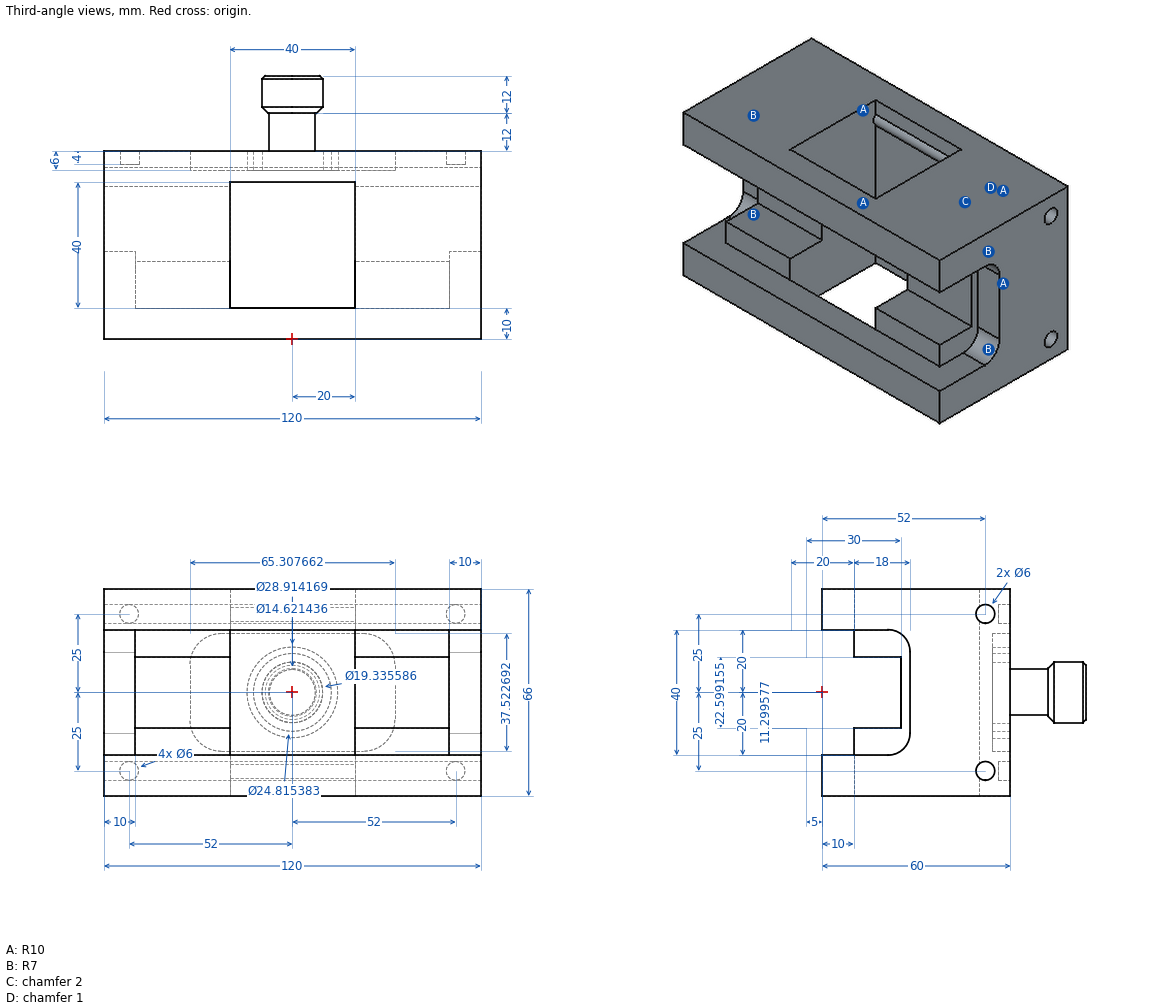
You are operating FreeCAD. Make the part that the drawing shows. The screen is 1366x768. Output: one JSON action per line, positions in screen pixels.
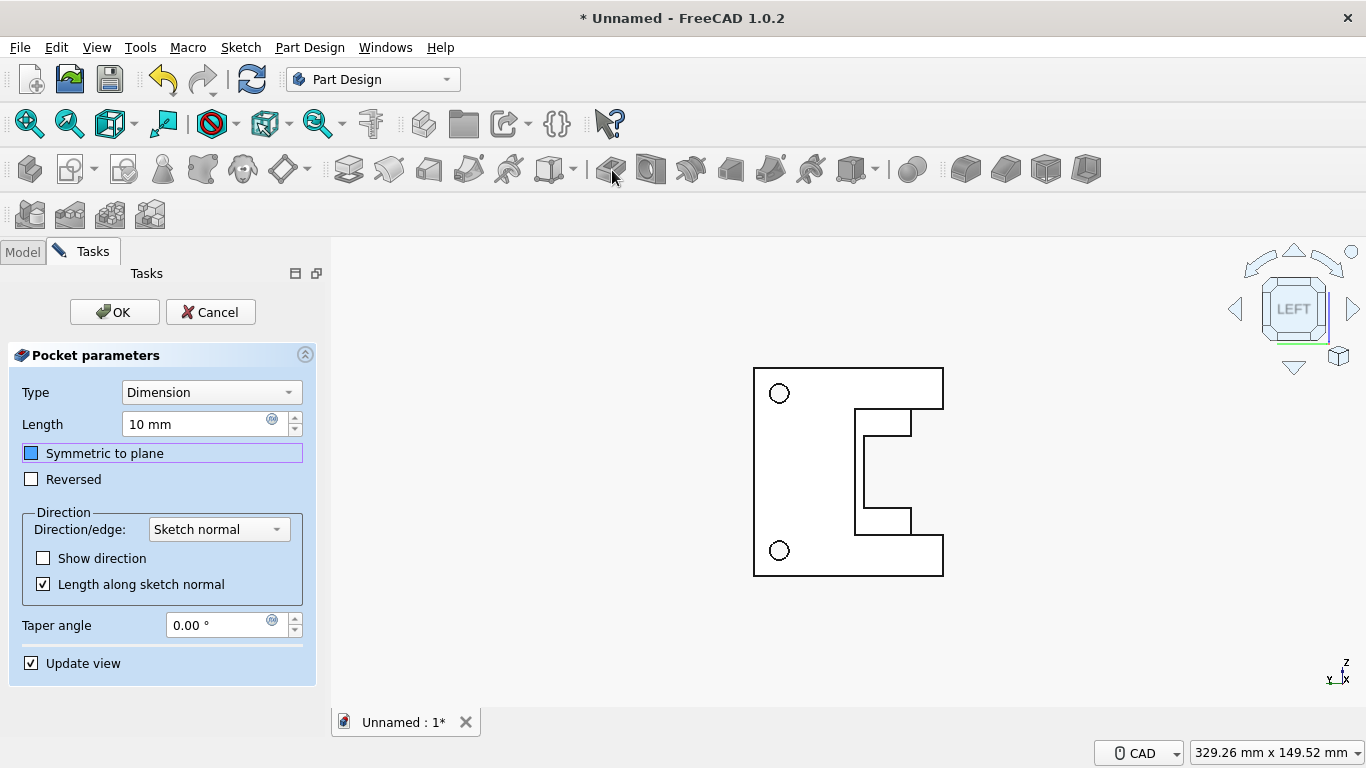
{"action": "left_click", "coordinate": [115, 312]}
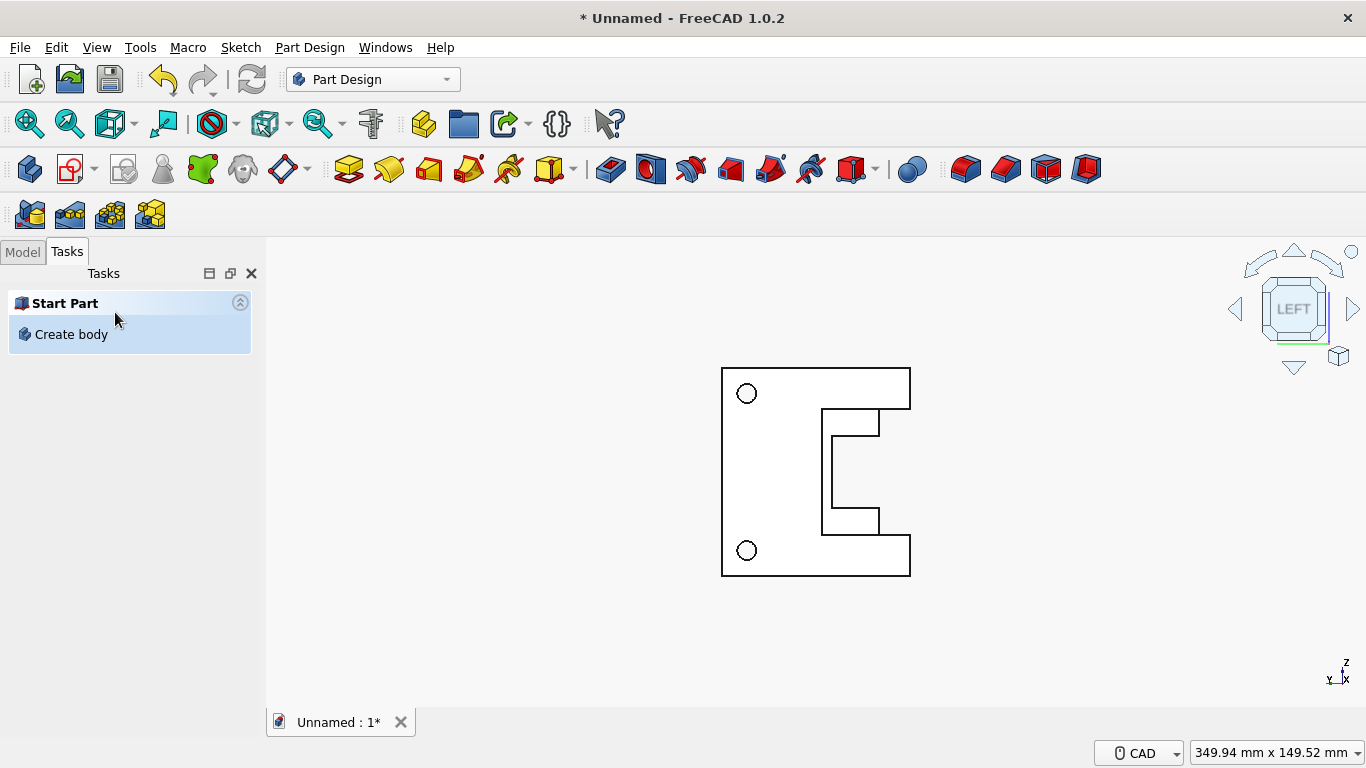
{"action": "left_click", "coordinate": [30, 124]}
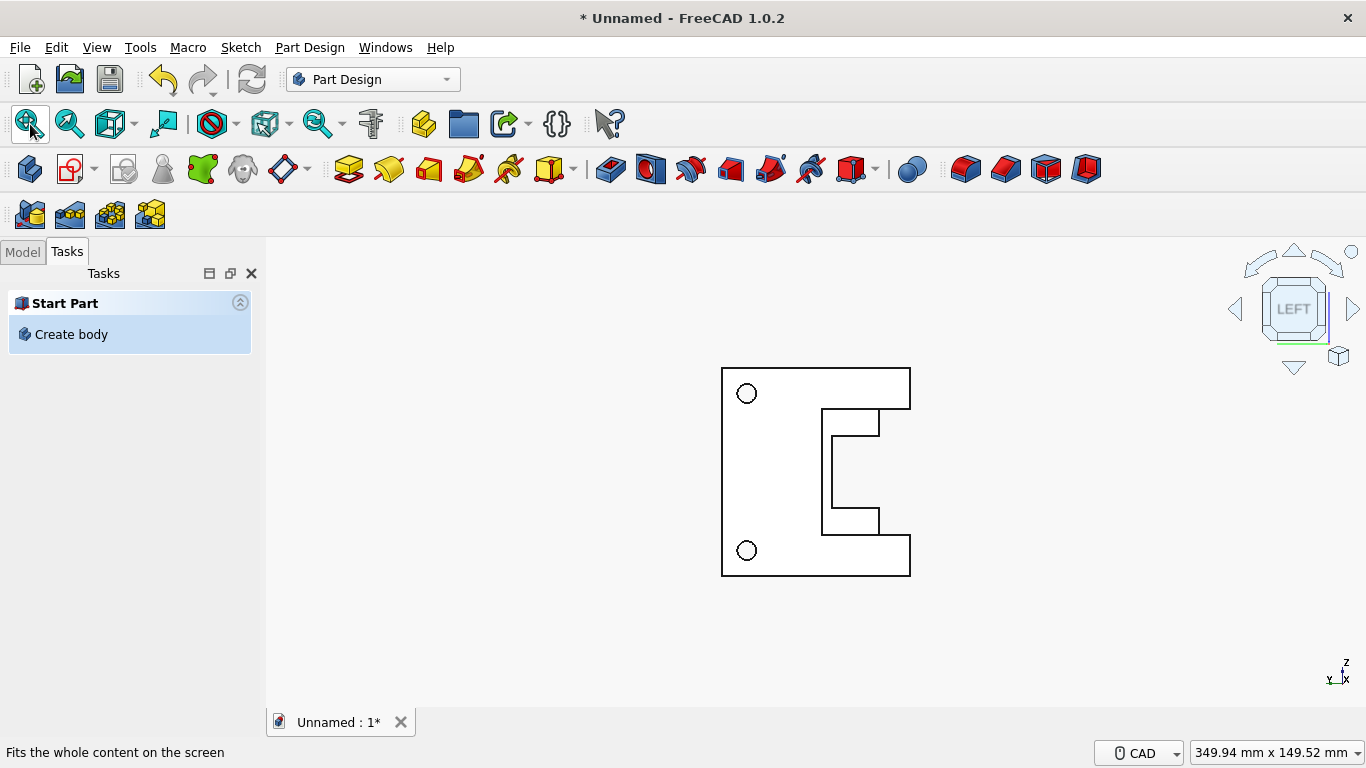
{"action": "key", "text": "4"}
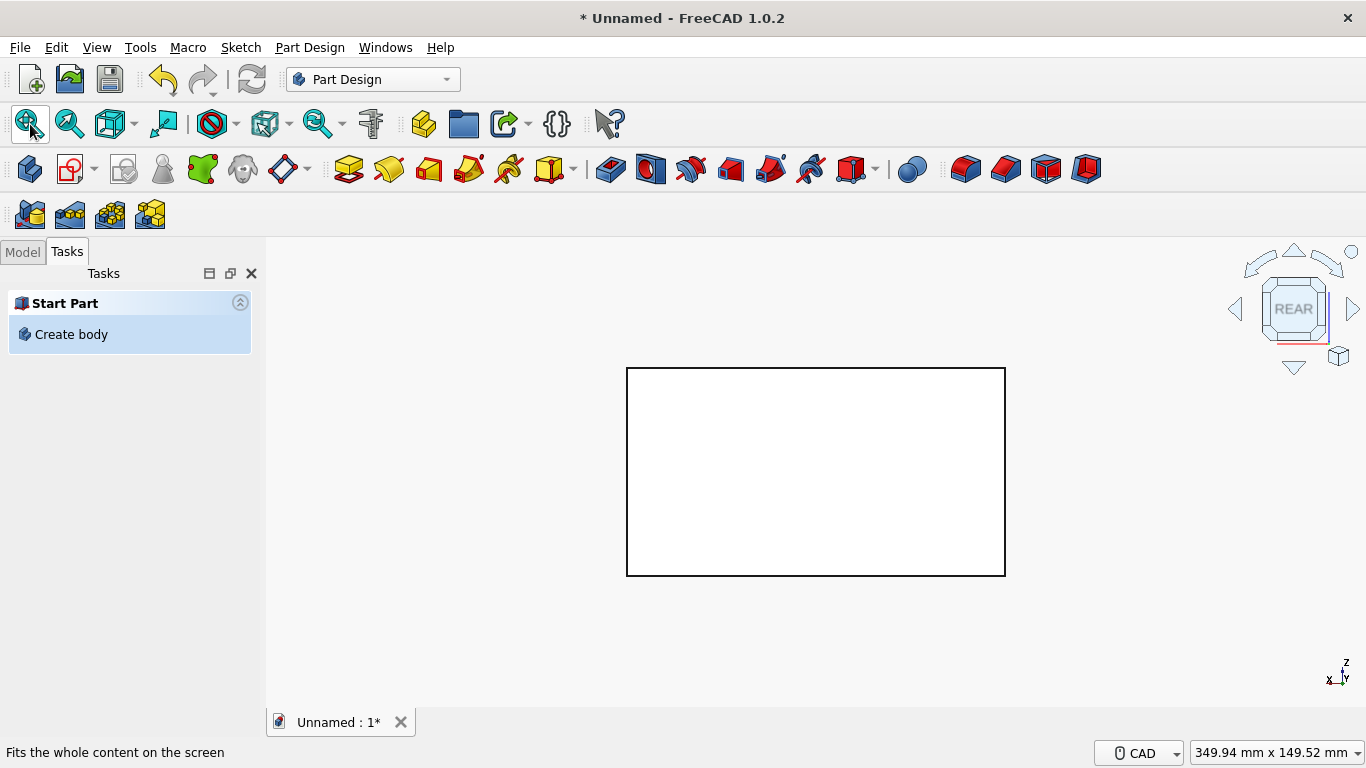
{"action": "left_click", "coordinate": [30, 124]}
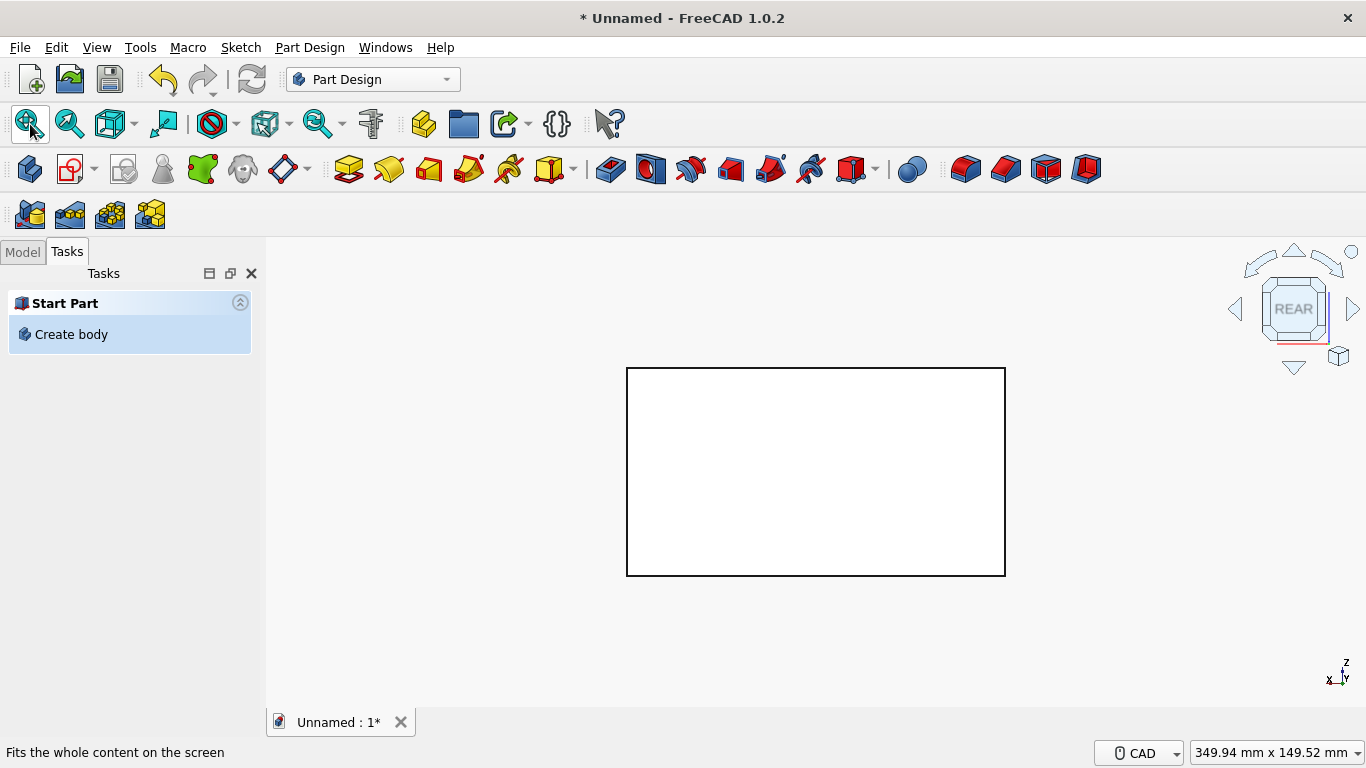
{"action": "left_click", "coordinate": [762, 471]}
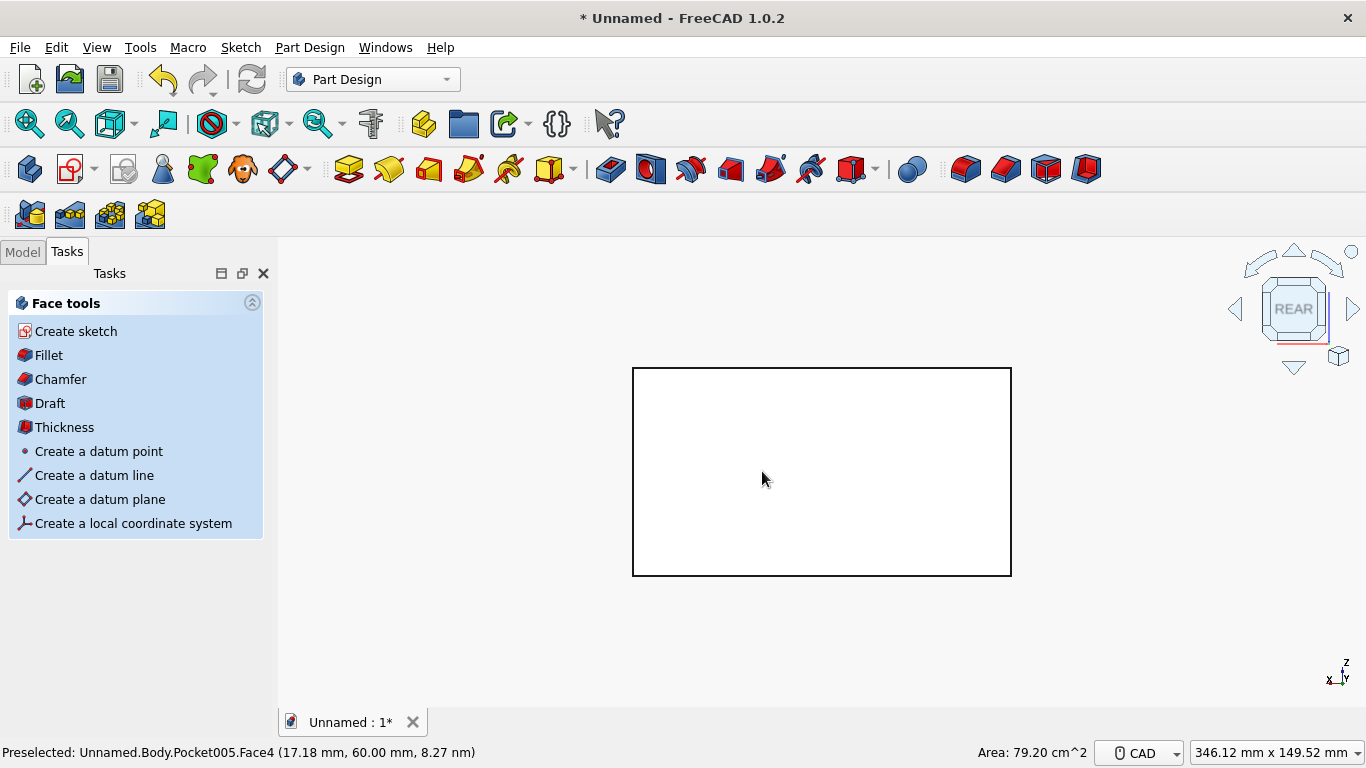
{"action": "left_click", "coordinate": [70, 170]}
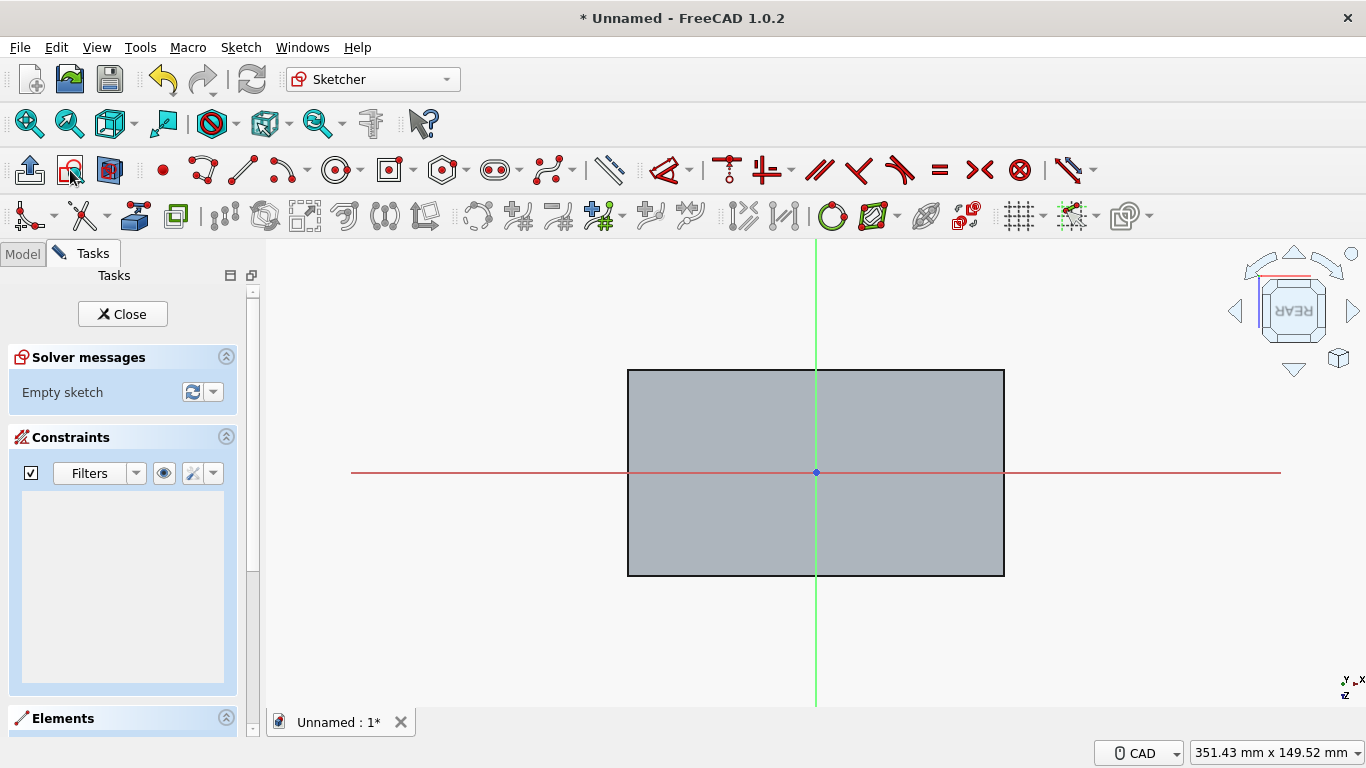
{"action": "scroll", "coordinate": [856, 473], "scroll_direction": "up", "scroll_amount": 5}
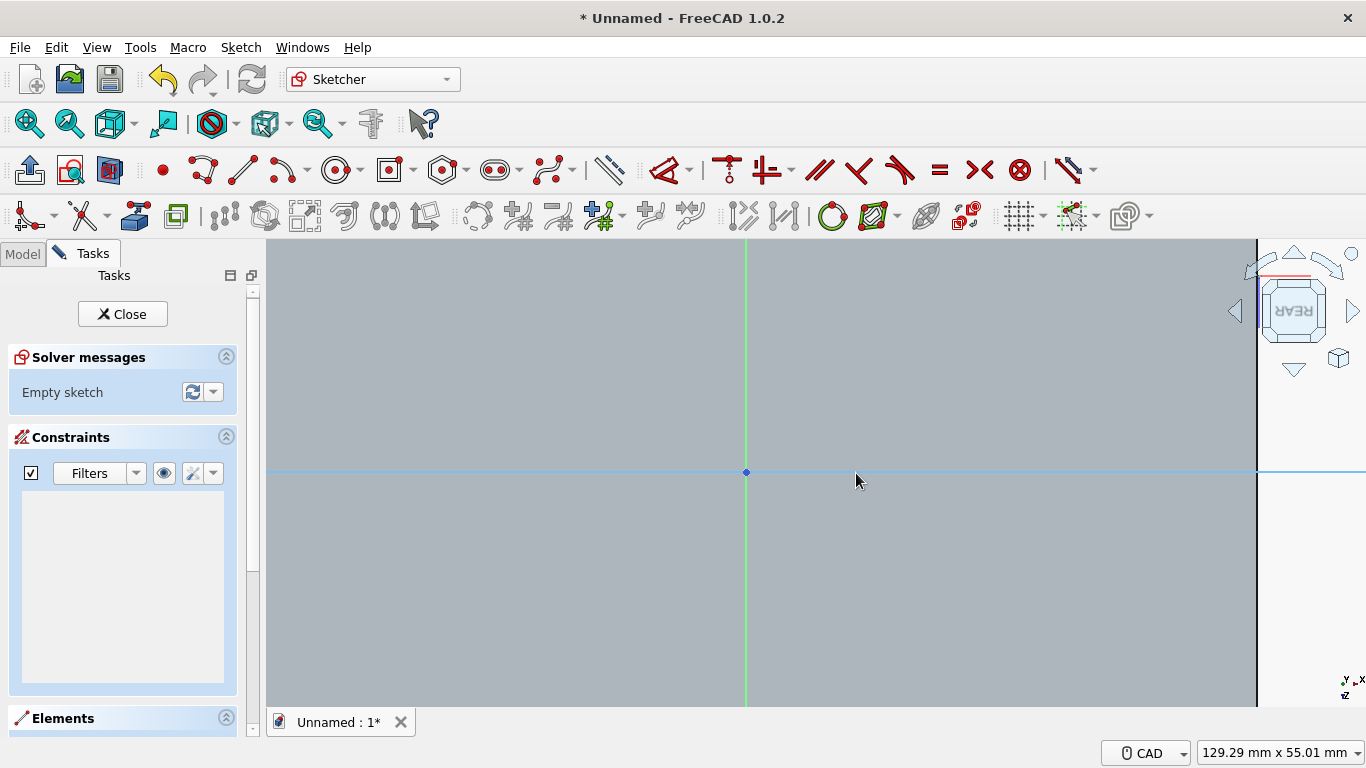
{"action": "left_click", "coordinate": [390, 170]}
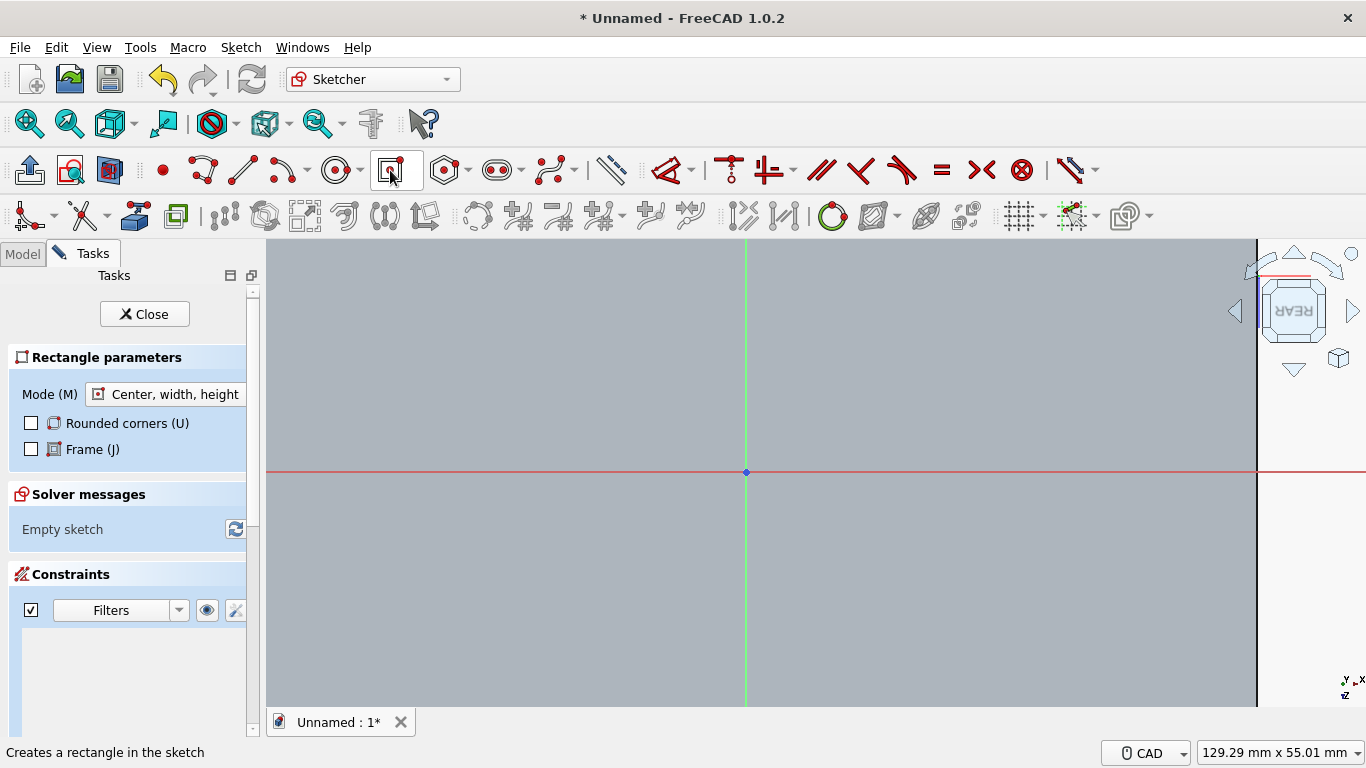
{"action": "left_click", "coordinate": [746, 472]}
{"action": "mouse_move", "coordinate": [1024, 313]}